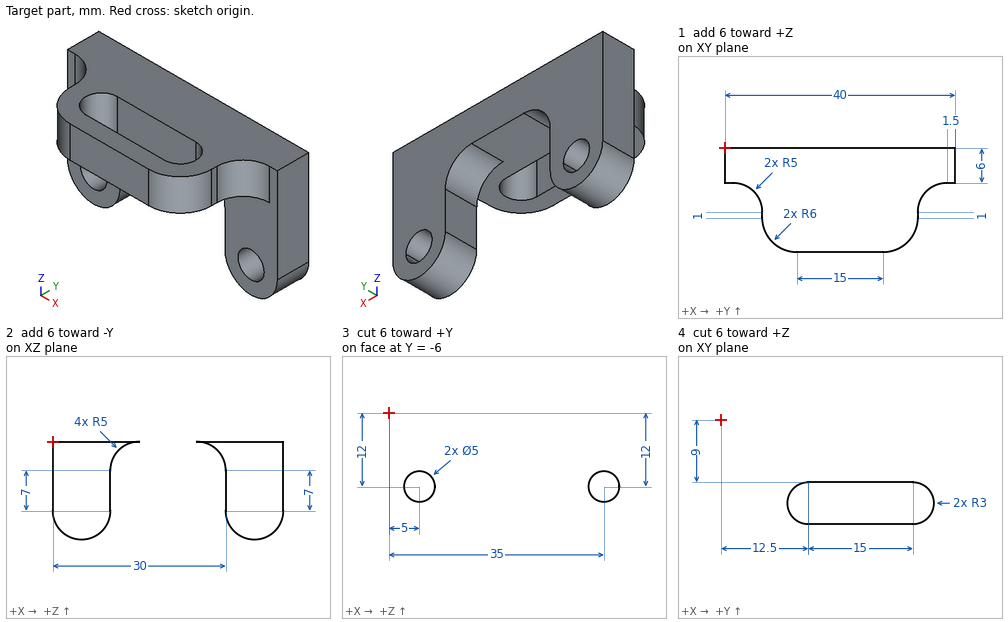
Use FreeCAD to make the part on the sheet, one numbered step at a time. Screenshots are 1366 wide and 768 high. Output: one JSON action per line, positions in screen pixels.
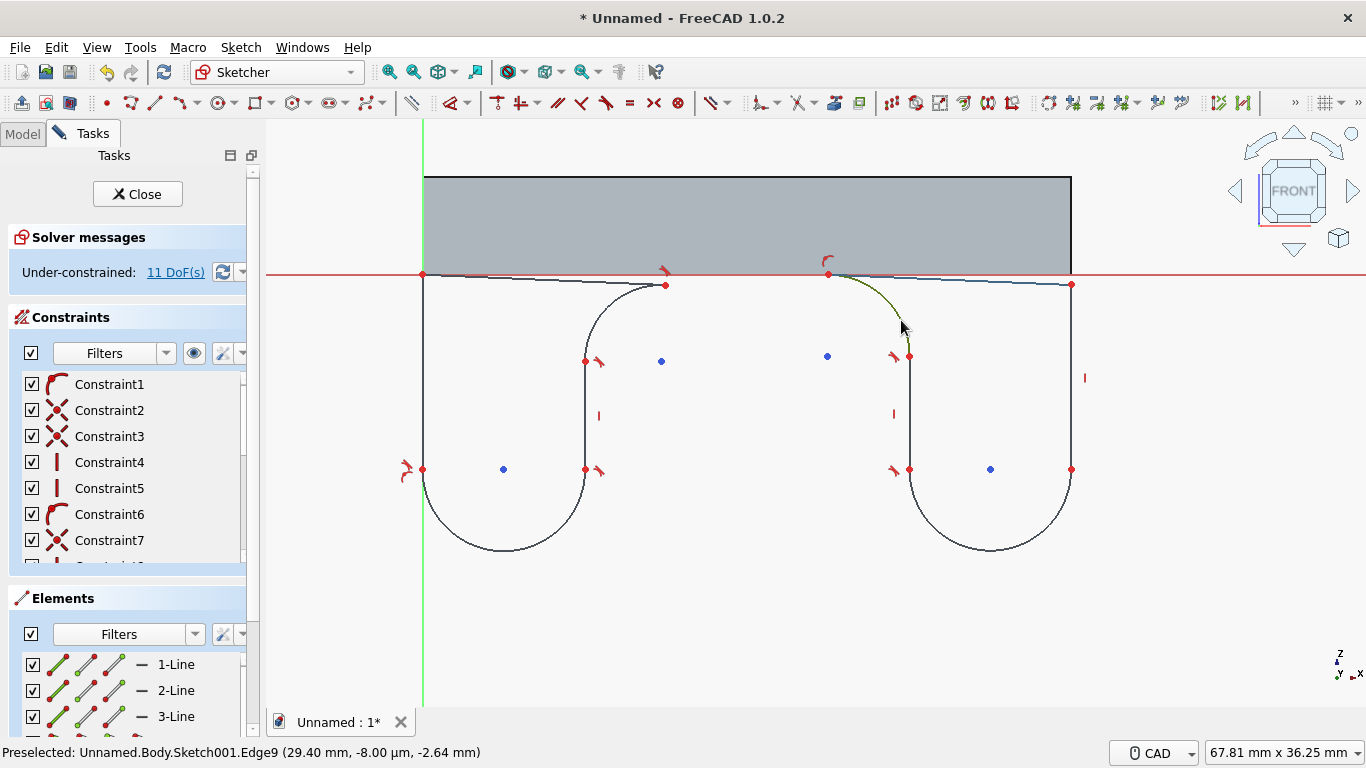
{"action": "key", "text": "t"}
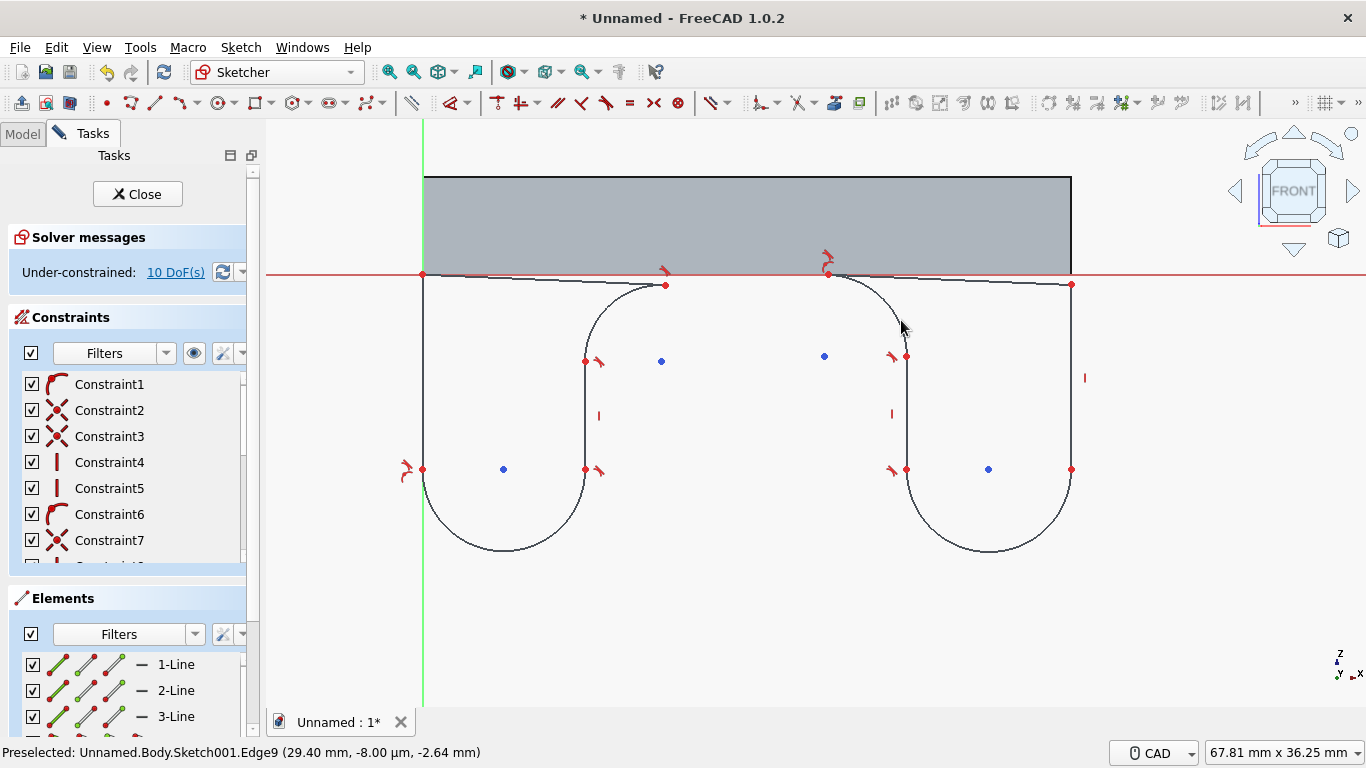
{"action": "left_click", "coordinate": [1071, 340]}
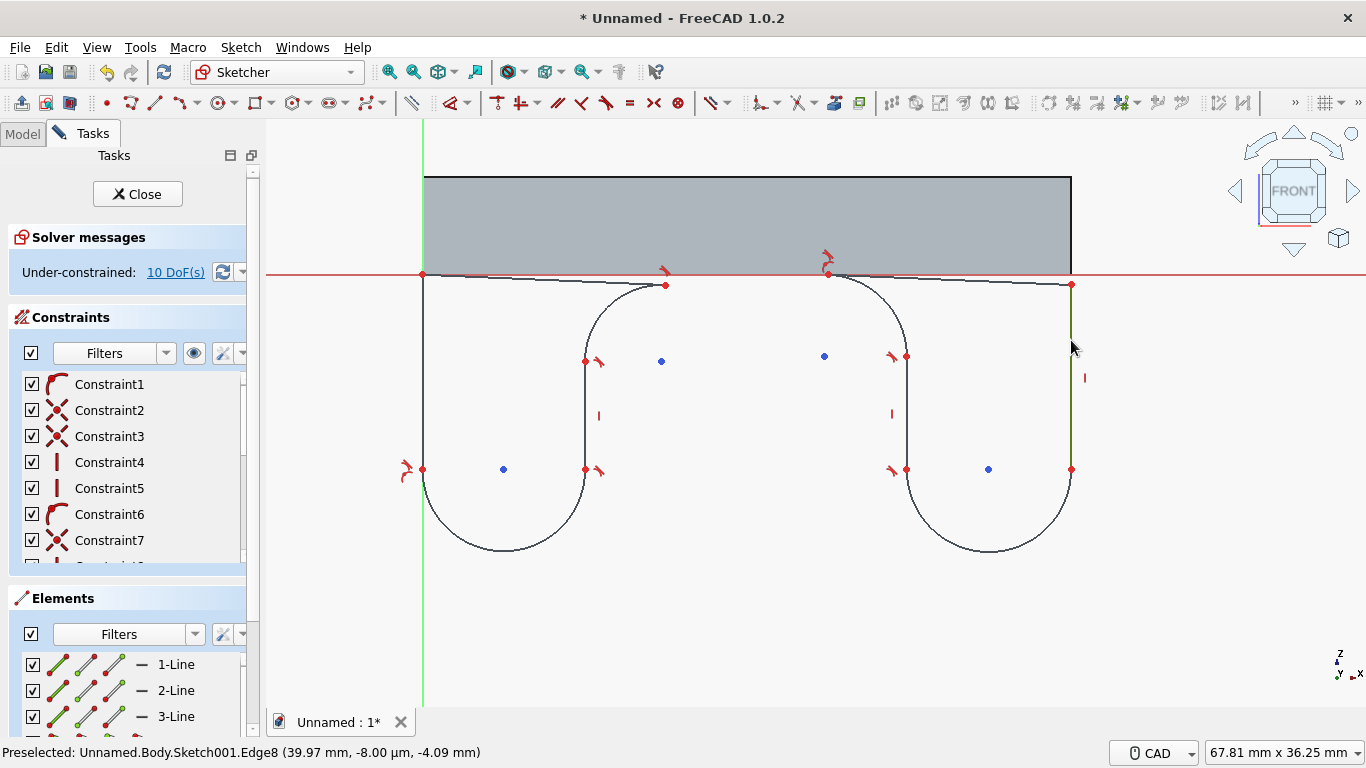
{"action": "left_click", "coordinate": [941, 536]}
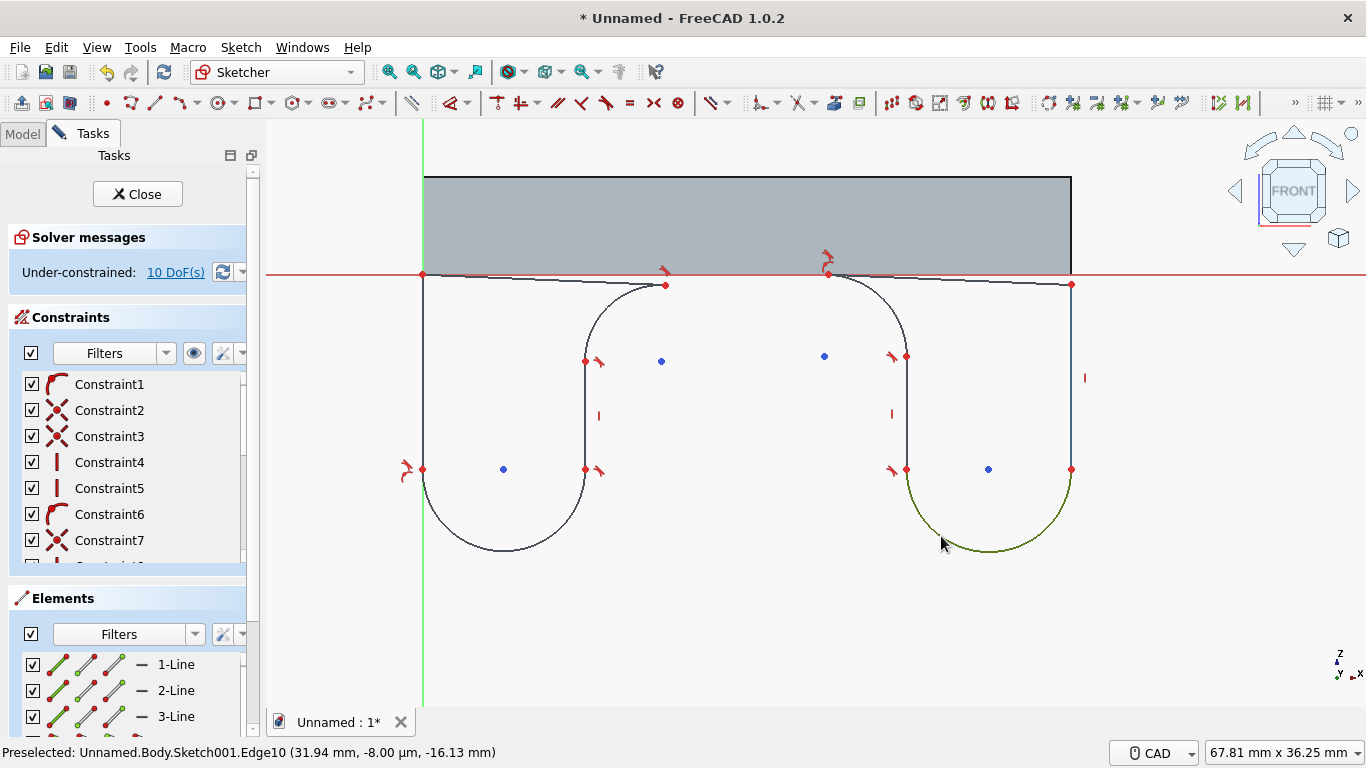
{"action": "key", "text": "t"}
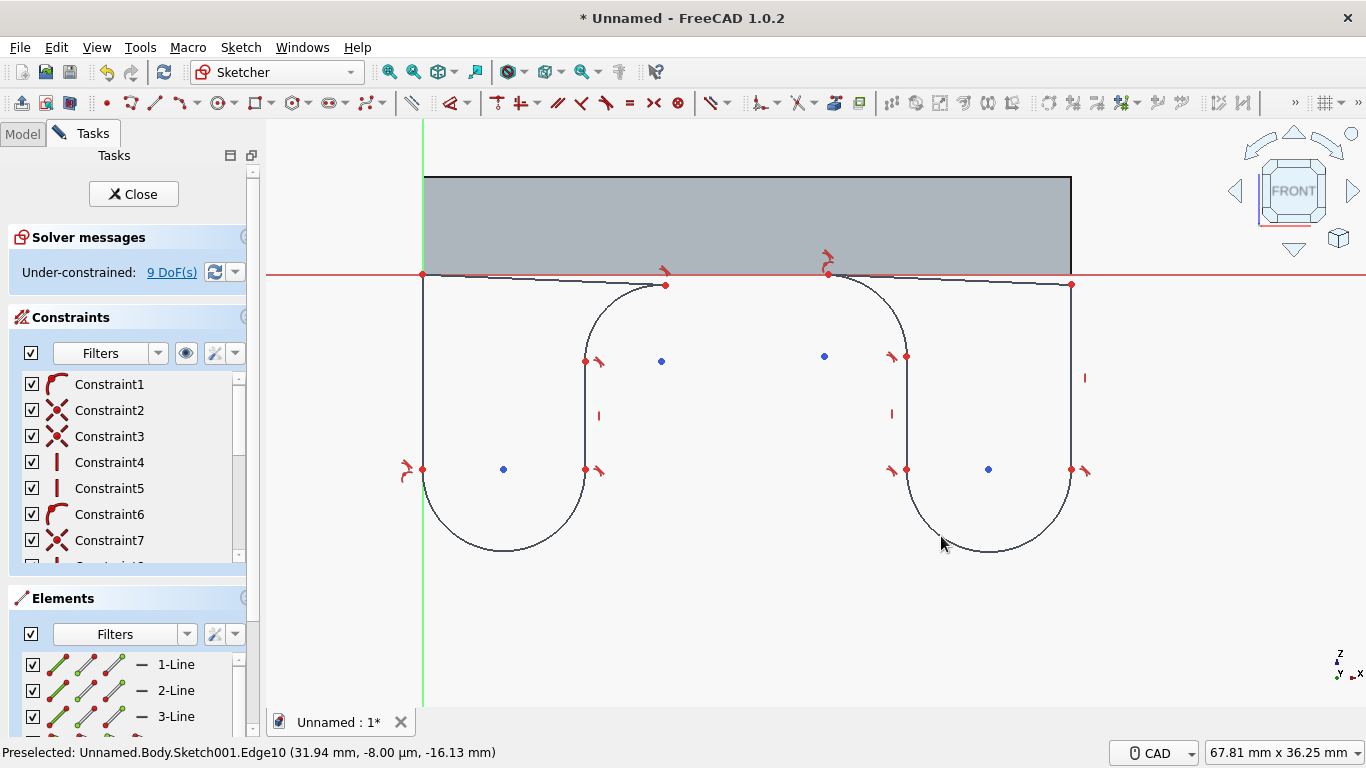
{"action": "left_click", "coordinate": [495, 278]}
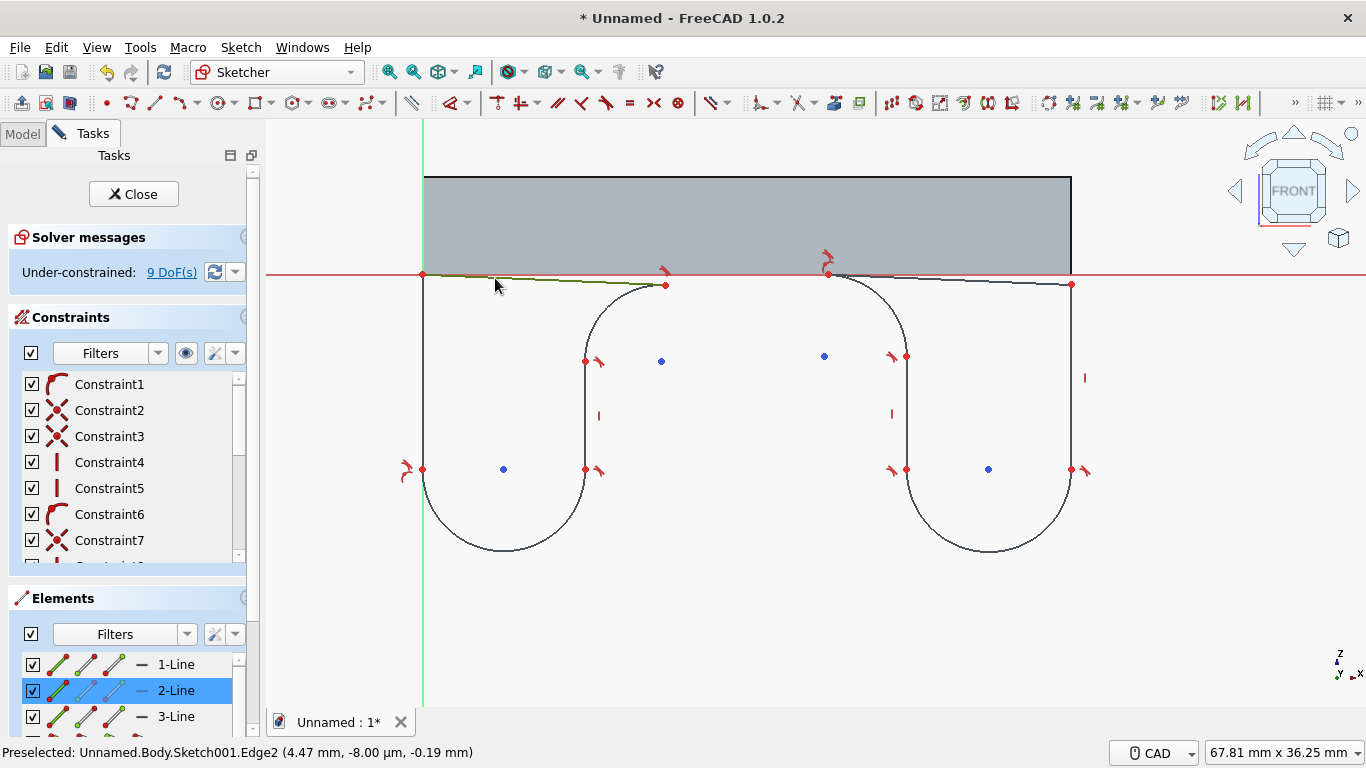
{"action": "key", "text": "h"}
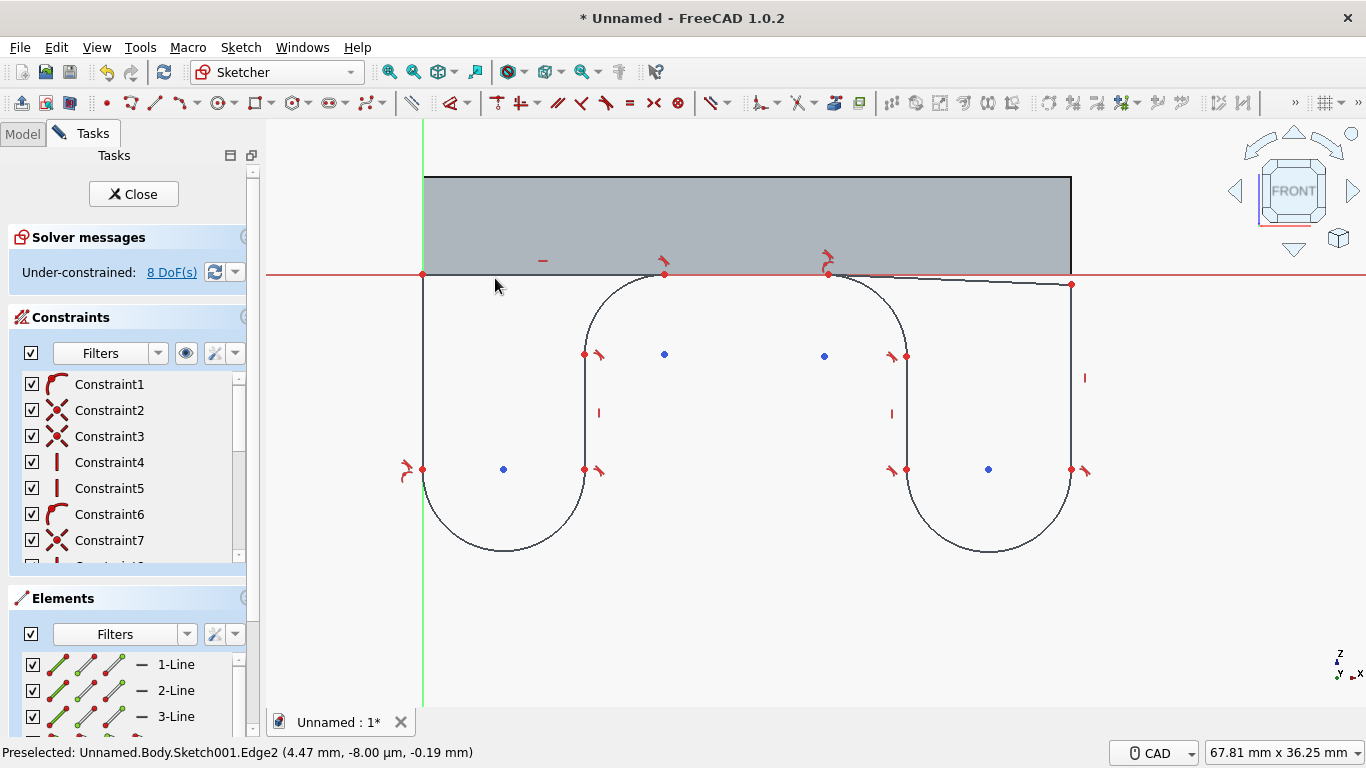
{"action": "left_click", "coordinate": [901, 278]}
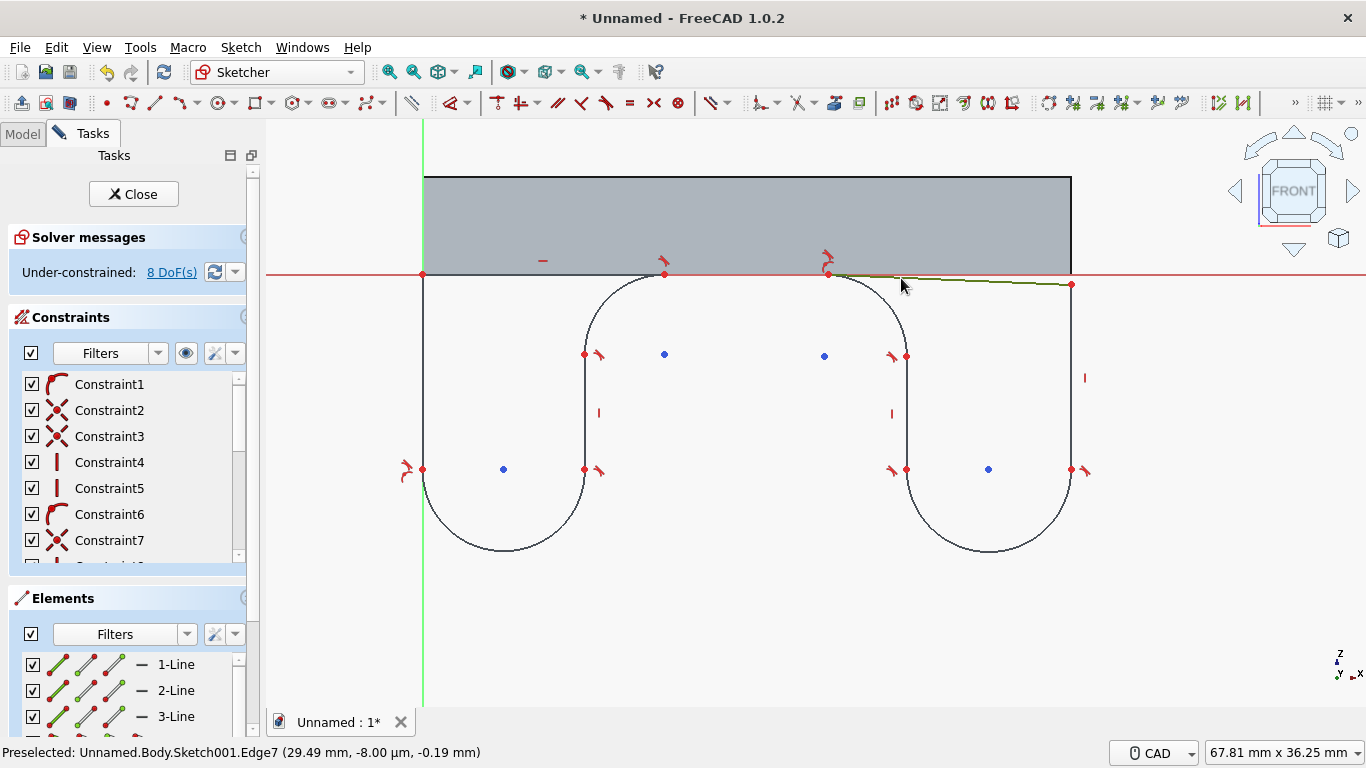
{"action": "key", "text": "h"}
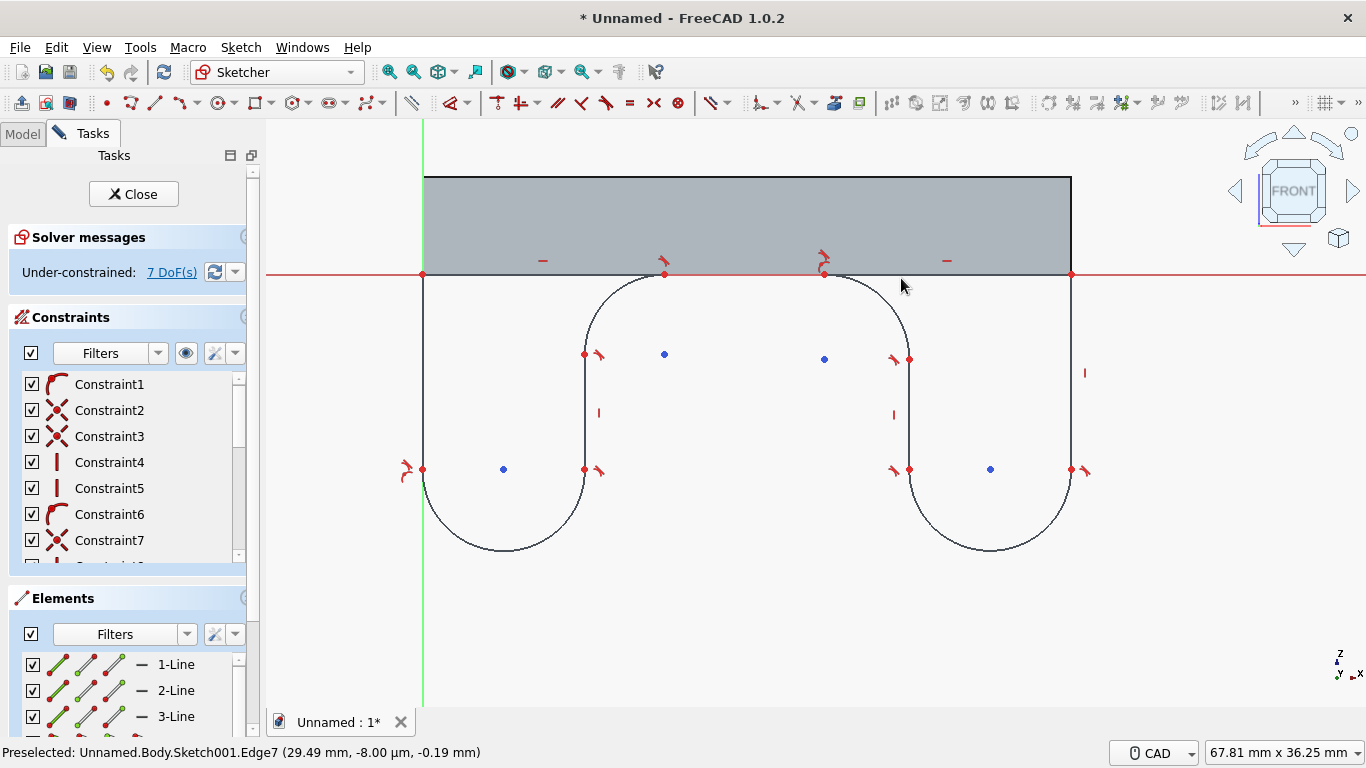
{"action": "left_click", "coordinate": [594, 318]}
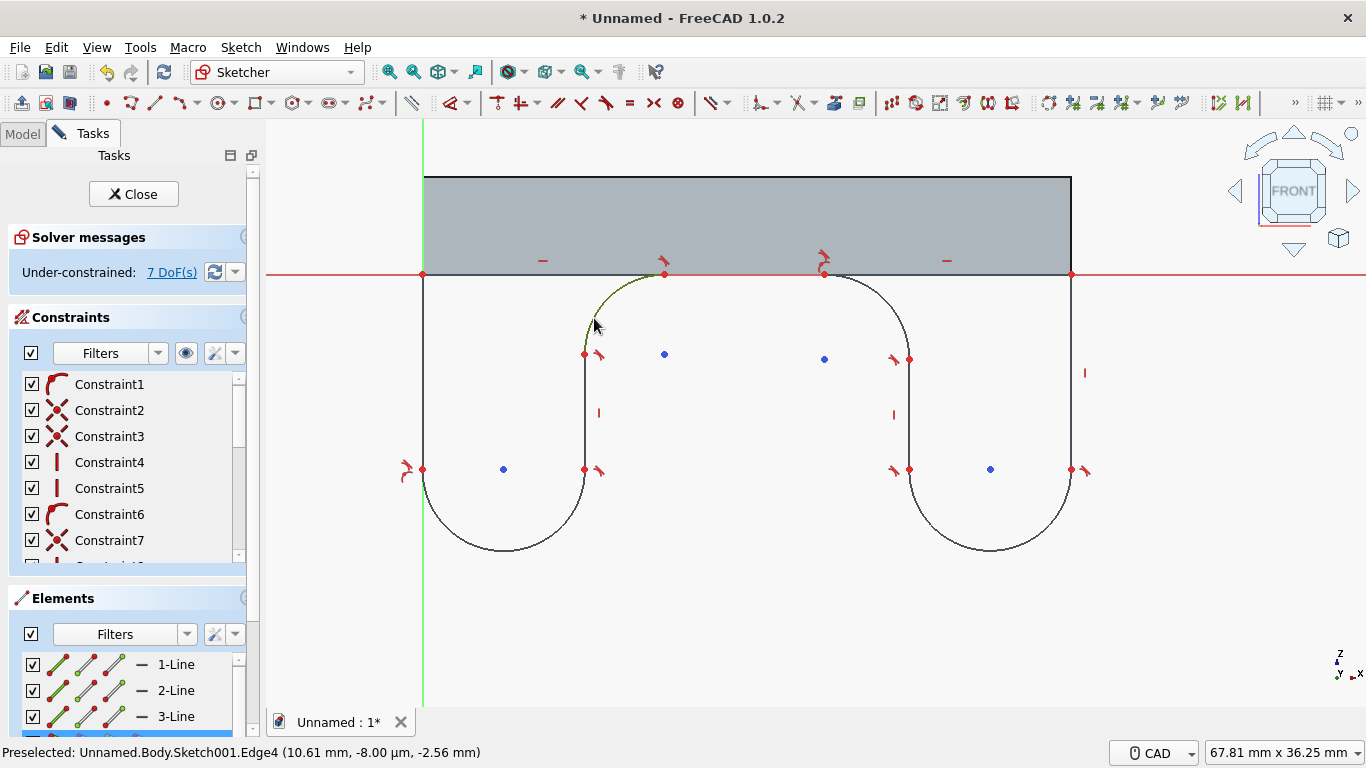
{"action": "left_click", "coordinate": [456, 536]}